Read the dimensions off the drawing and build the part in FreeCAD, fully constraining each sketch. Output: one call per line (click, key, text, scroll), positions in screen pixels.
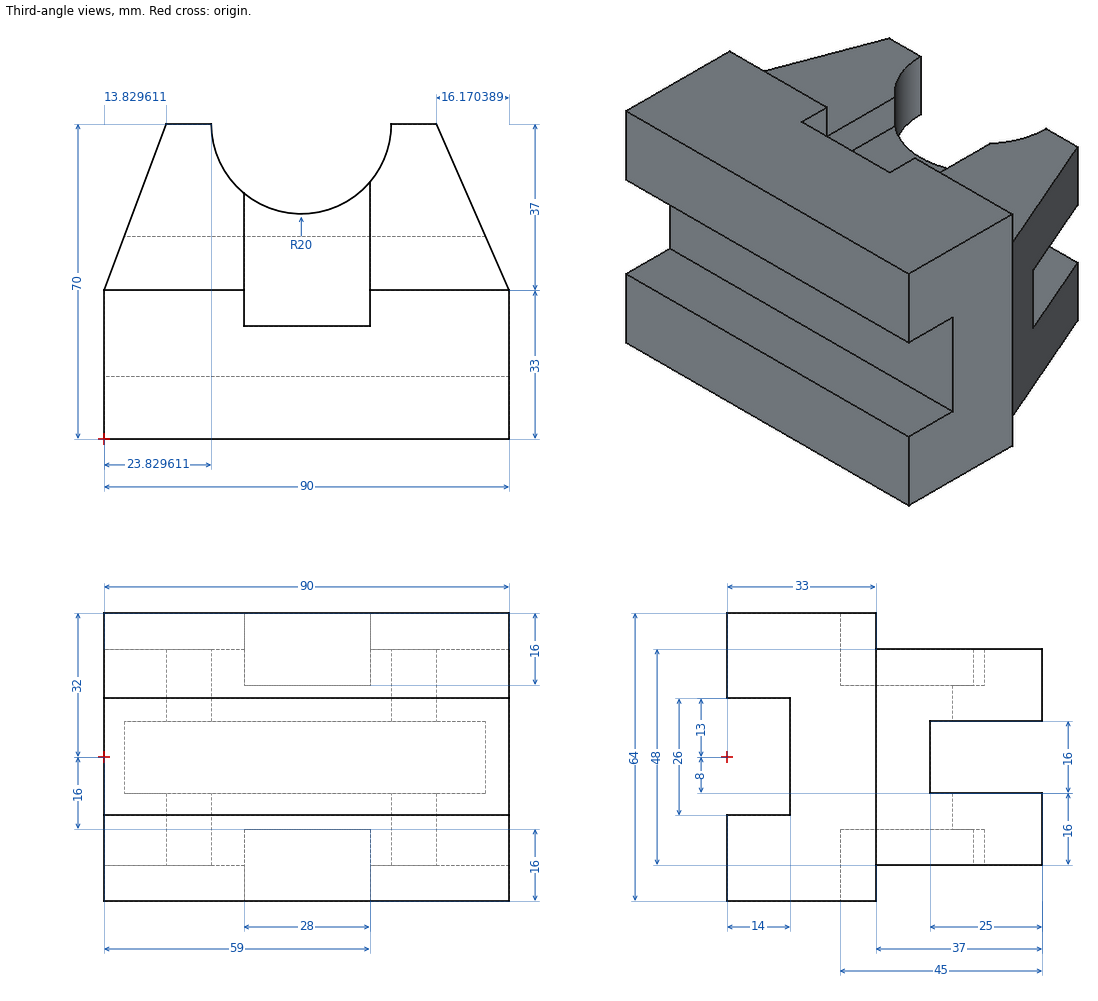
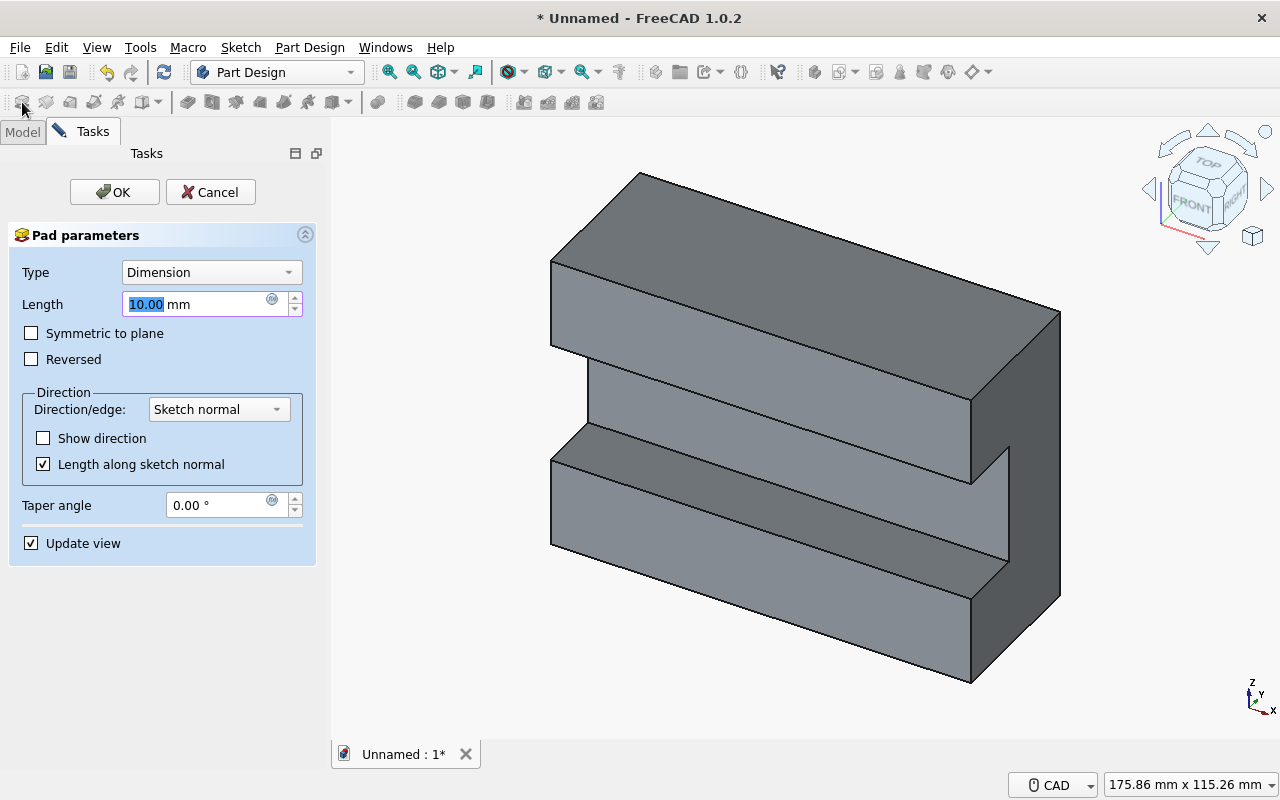
text(90)
key(Tab)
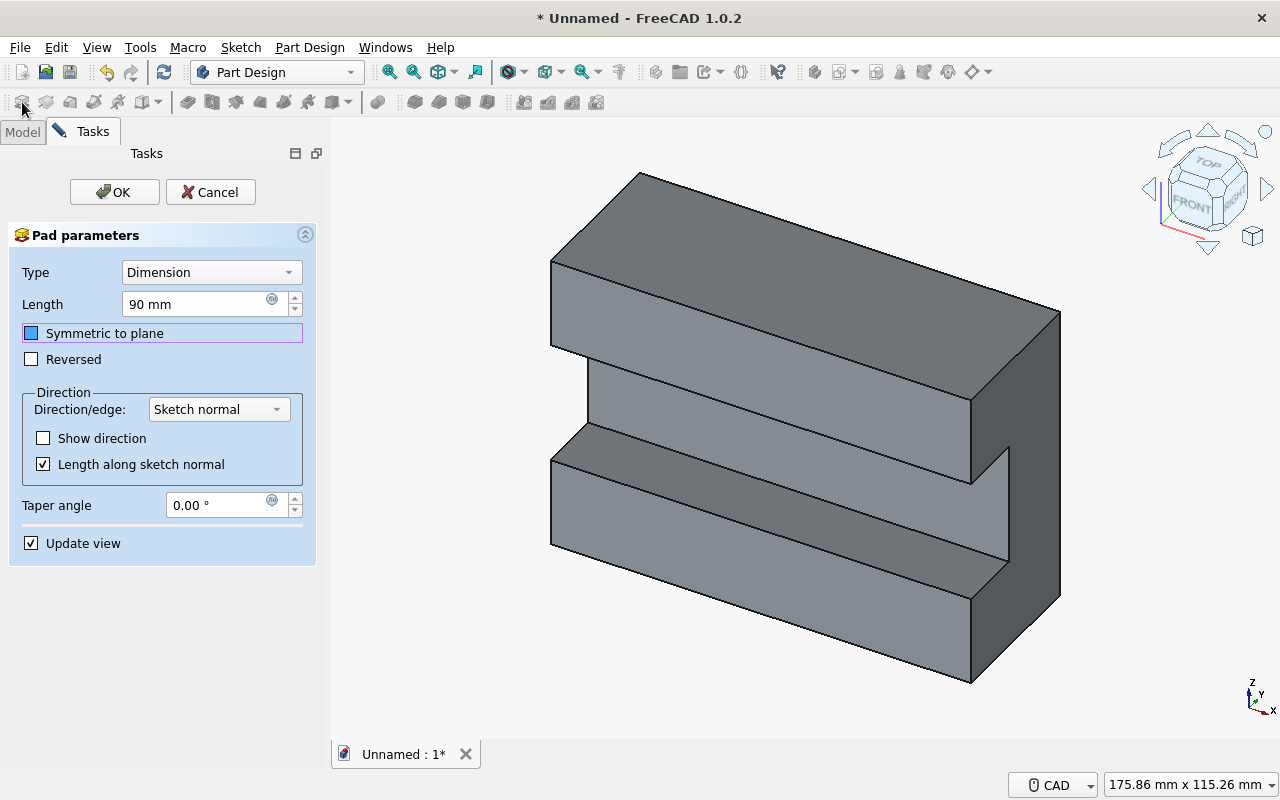
click(30, 359)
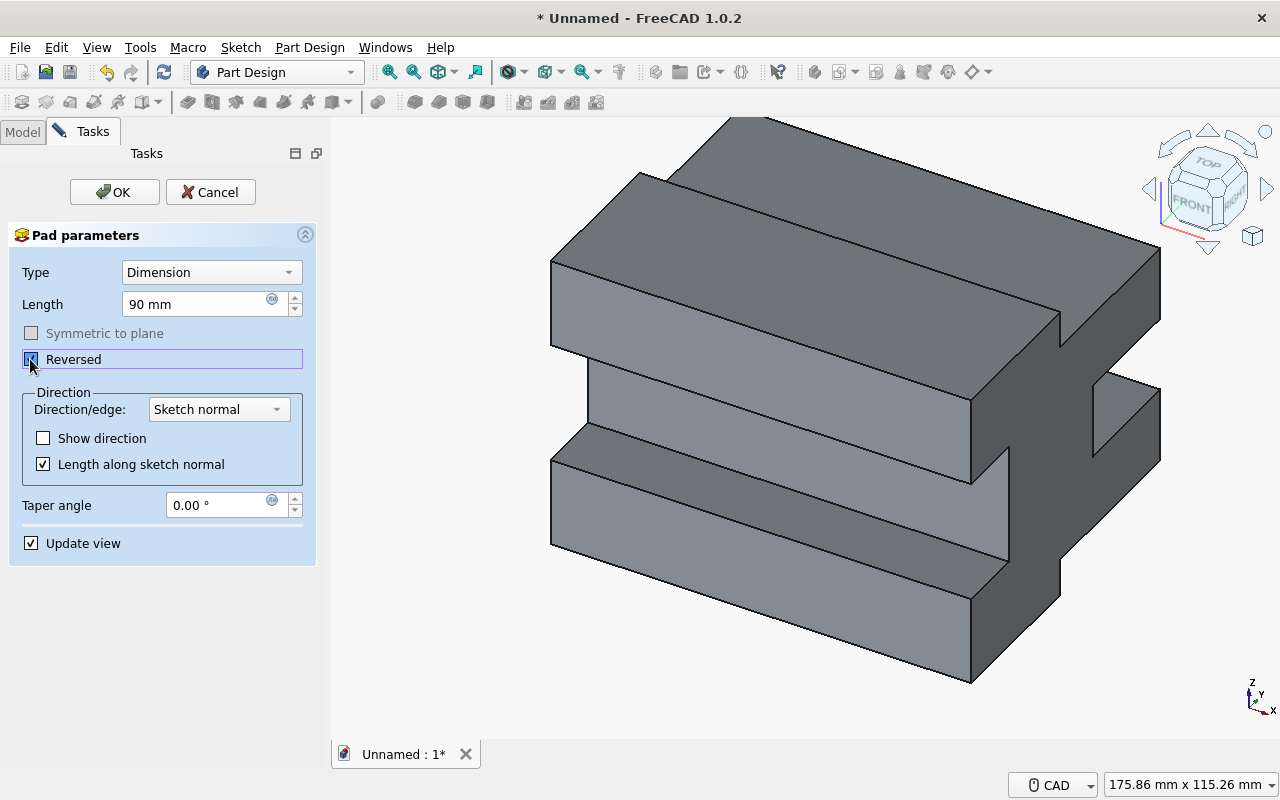
click(115, 192)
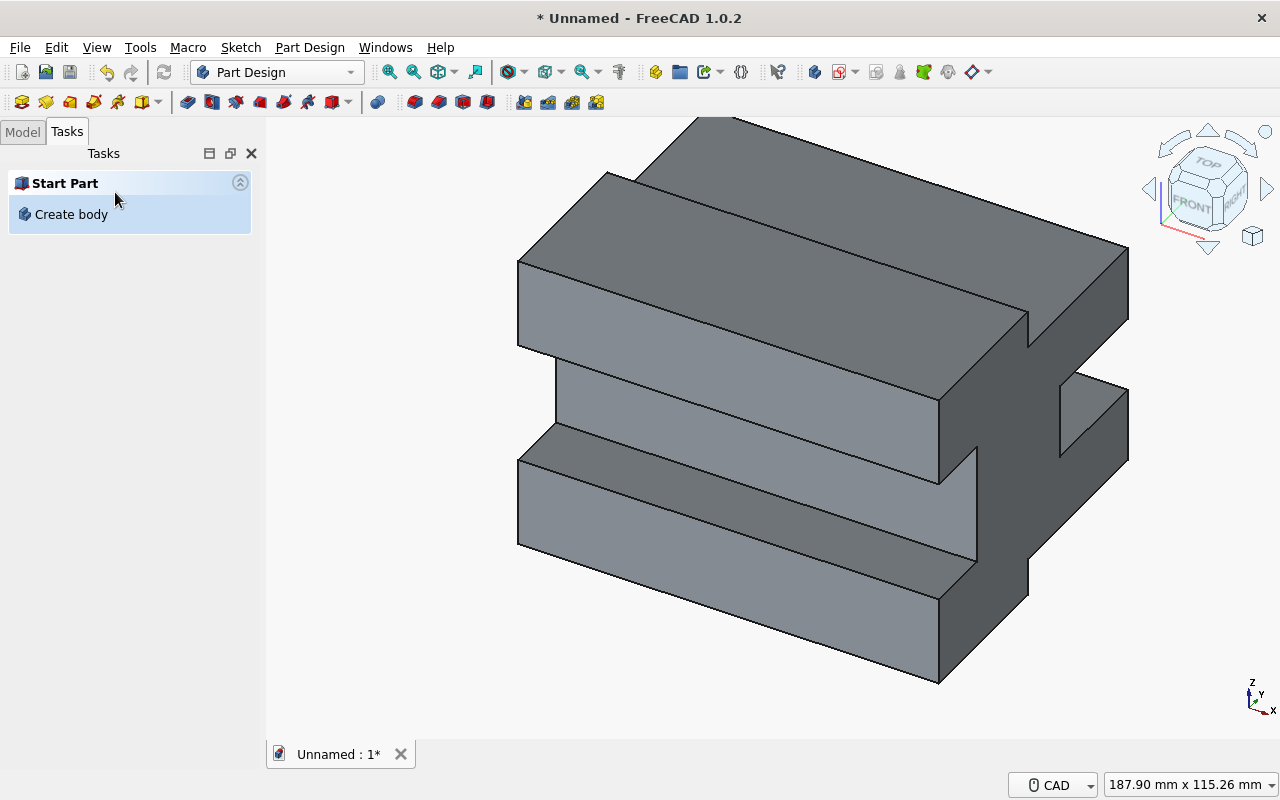
click(390, 72)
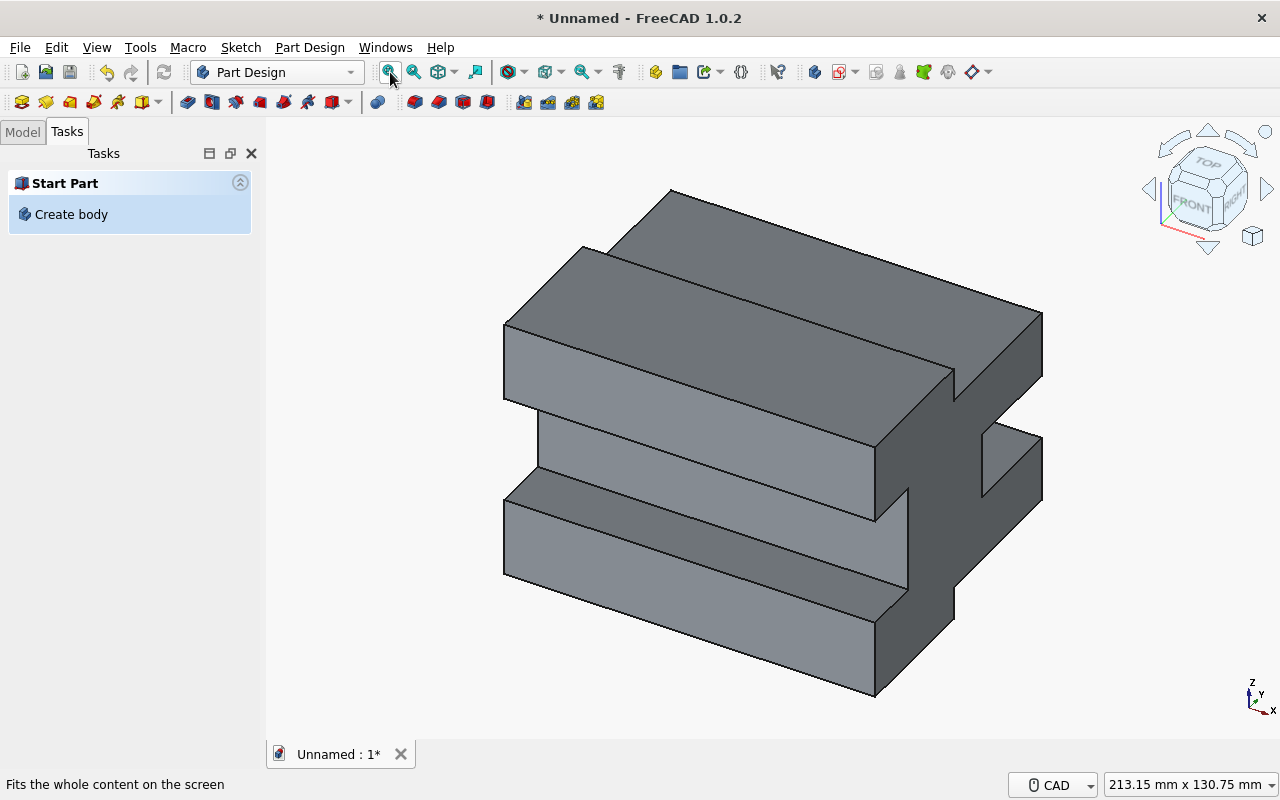
click(918, 330)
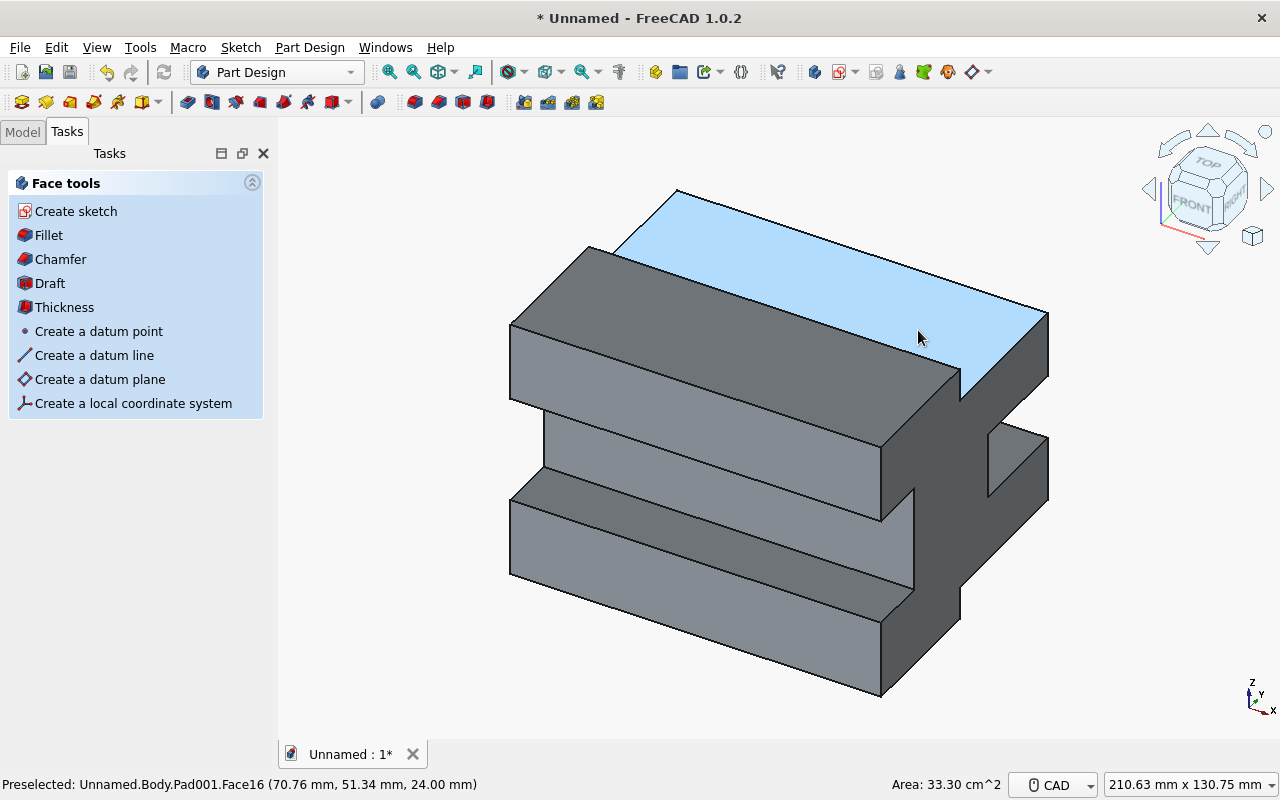
click(840, 72)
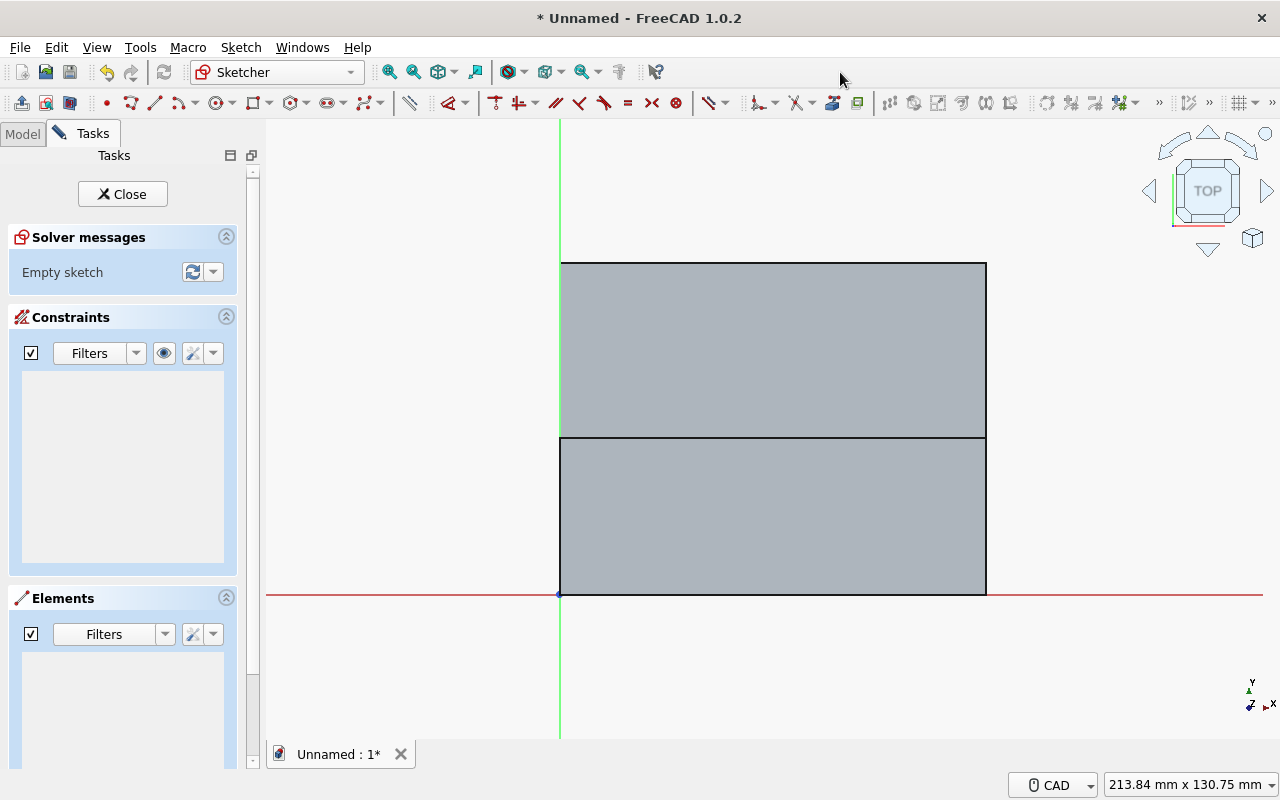
key(g)
key(m)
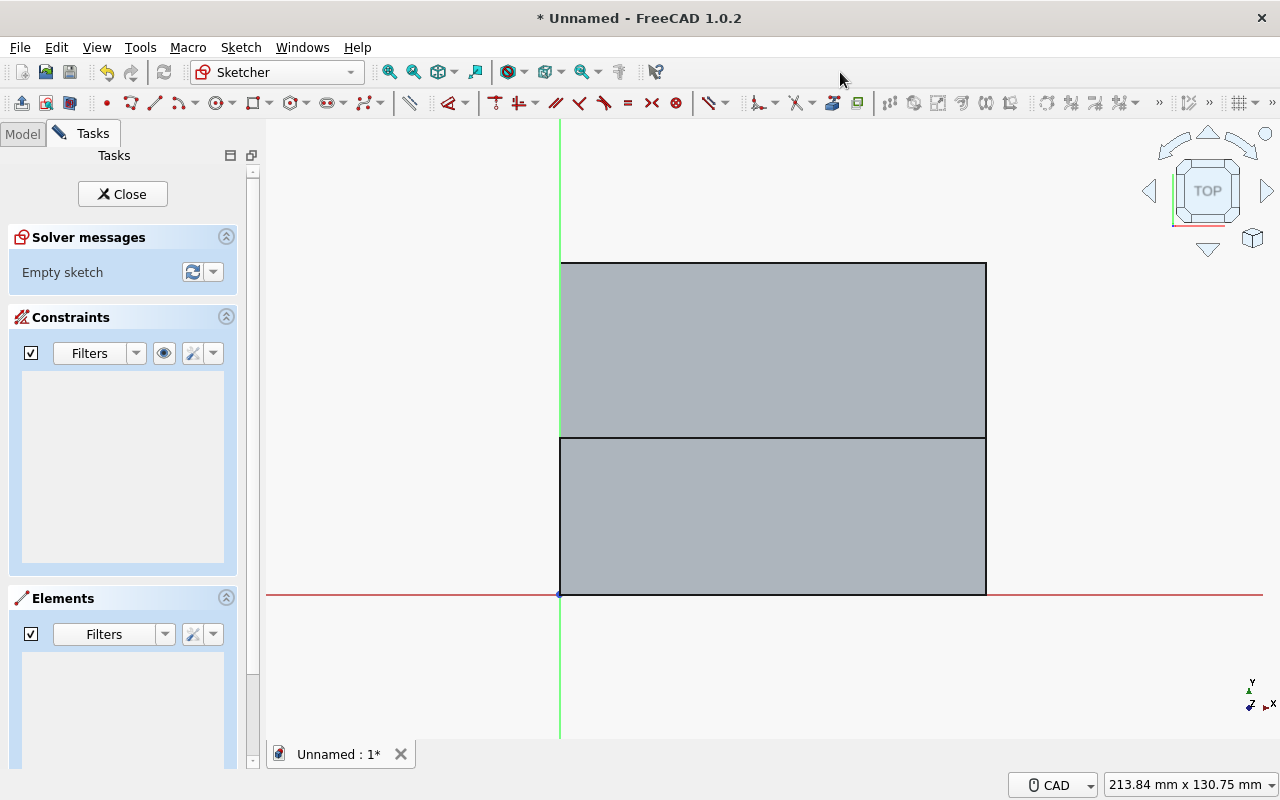
click(986, 438)
click(986, 263)
click(910, 263)
click(986, 439)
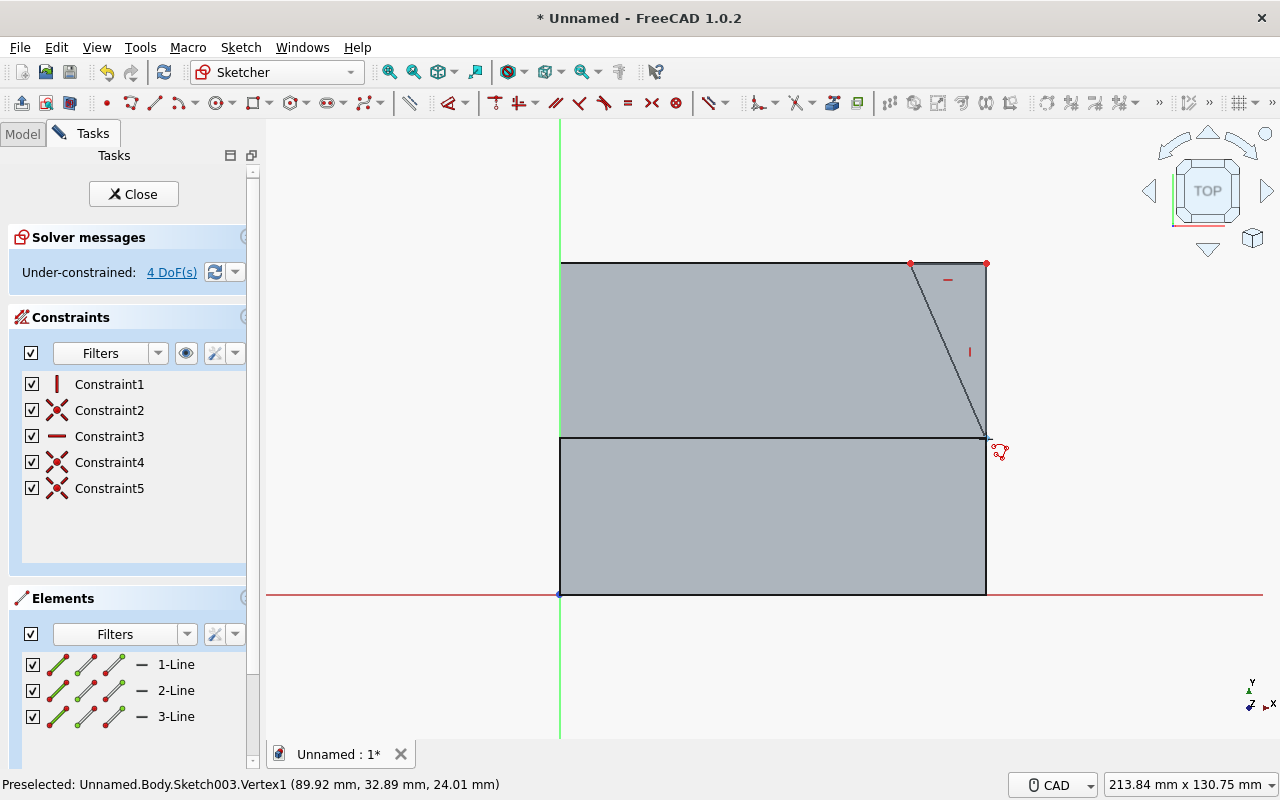
click(560, 438)
click(625, 263)
click(569, 263)
click(560, 439)
key(Escape)
key(Escape)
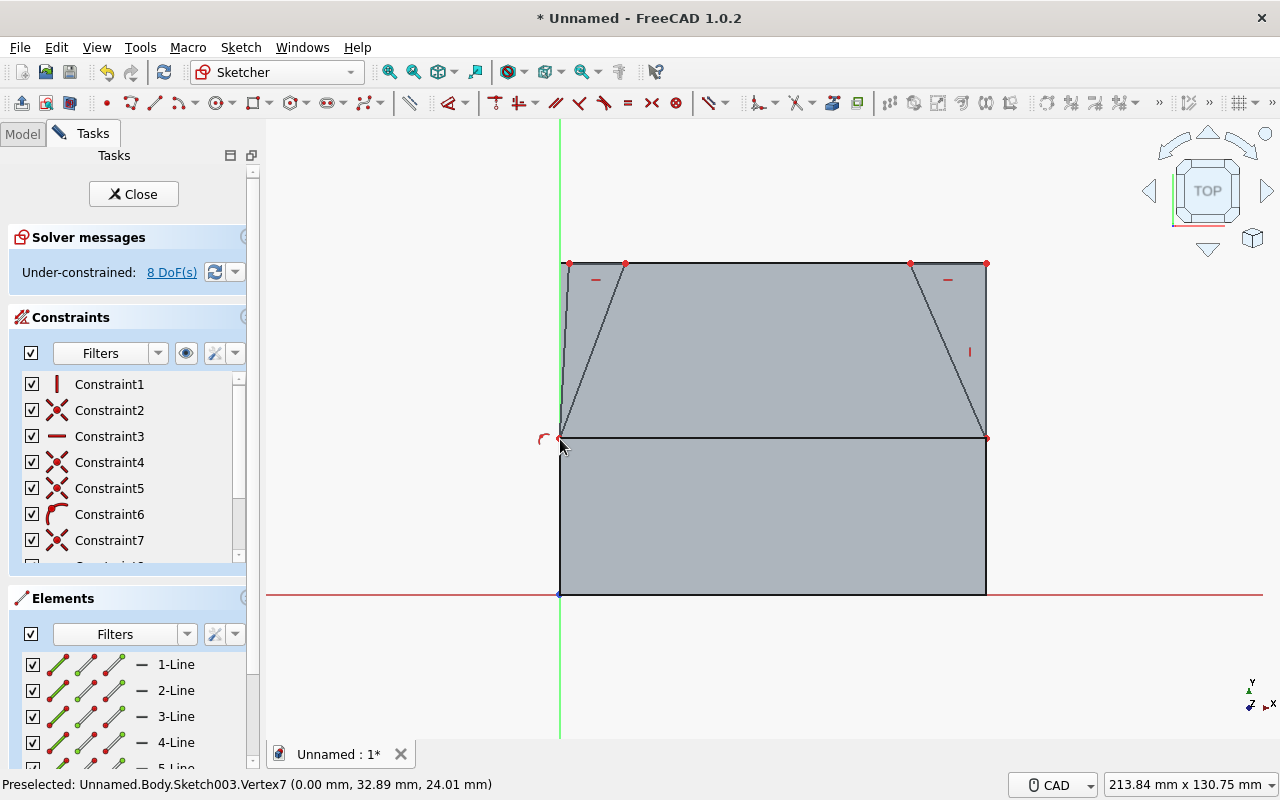
click(562, 387)